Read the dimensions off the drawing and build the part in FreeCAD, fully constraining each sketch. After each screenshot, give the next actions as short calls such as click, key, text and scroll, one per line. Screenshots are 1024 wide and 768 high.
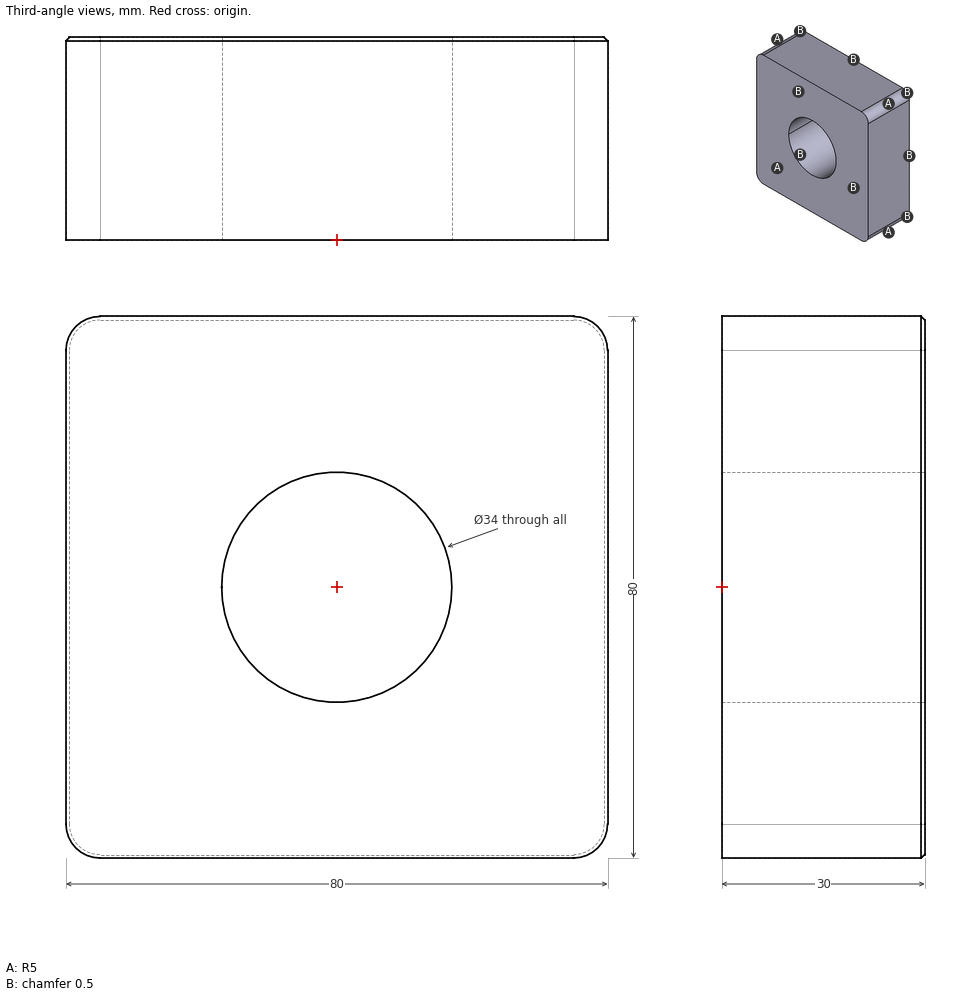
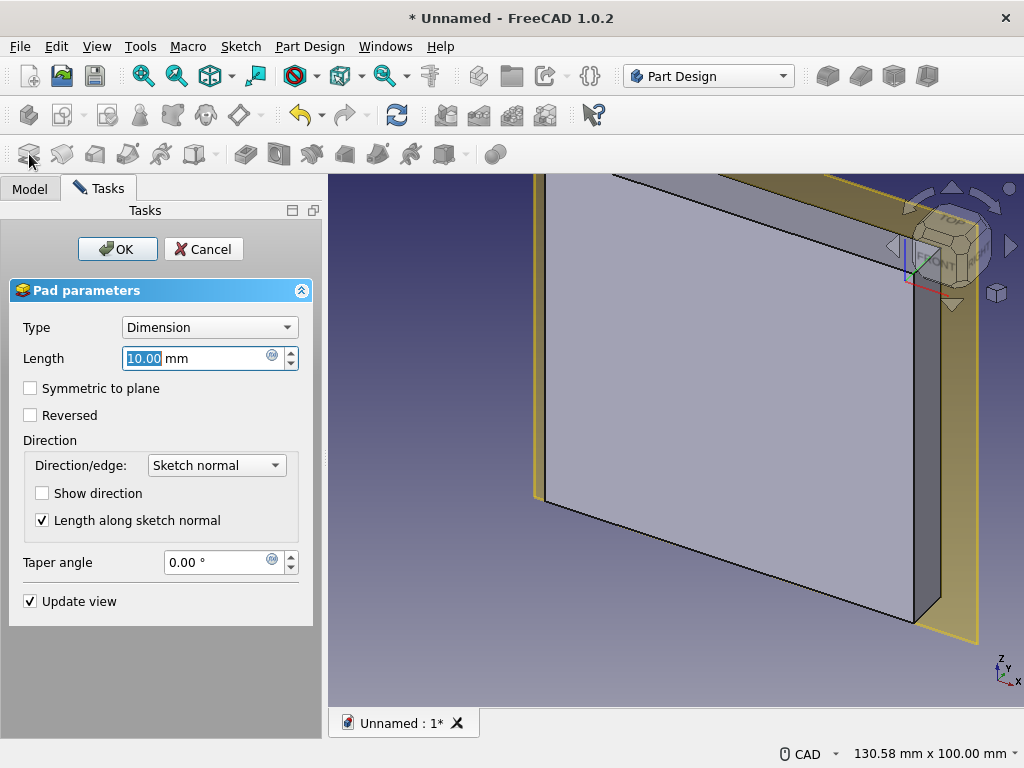
text(30)
key(Tab)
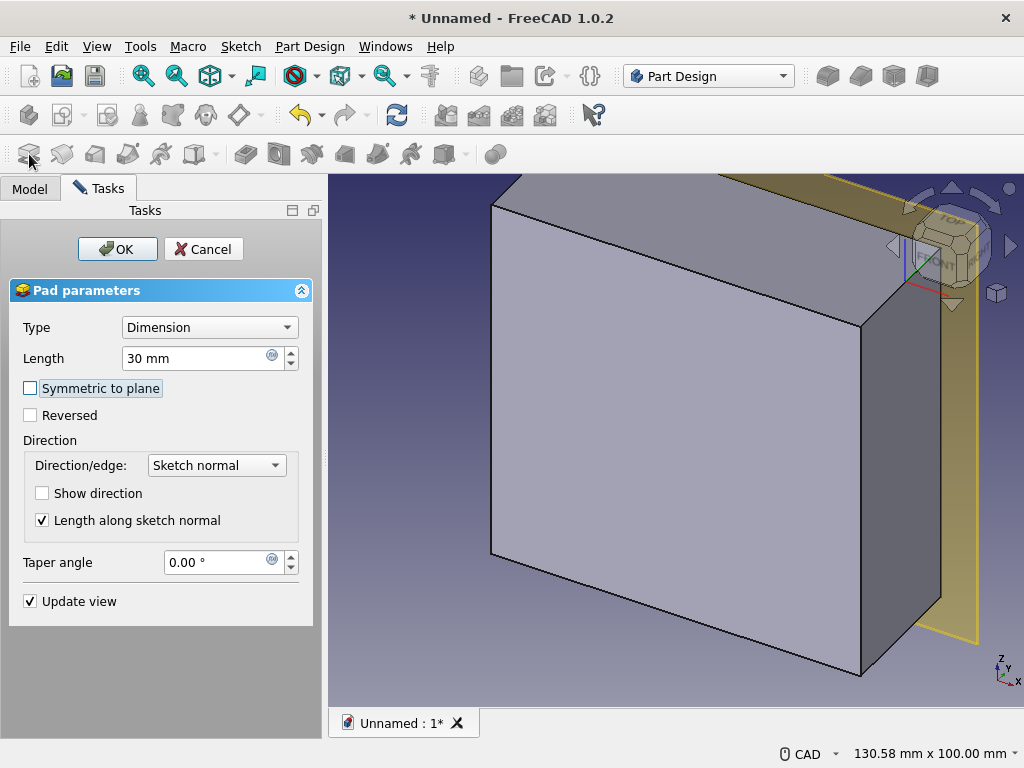
click(118, 249)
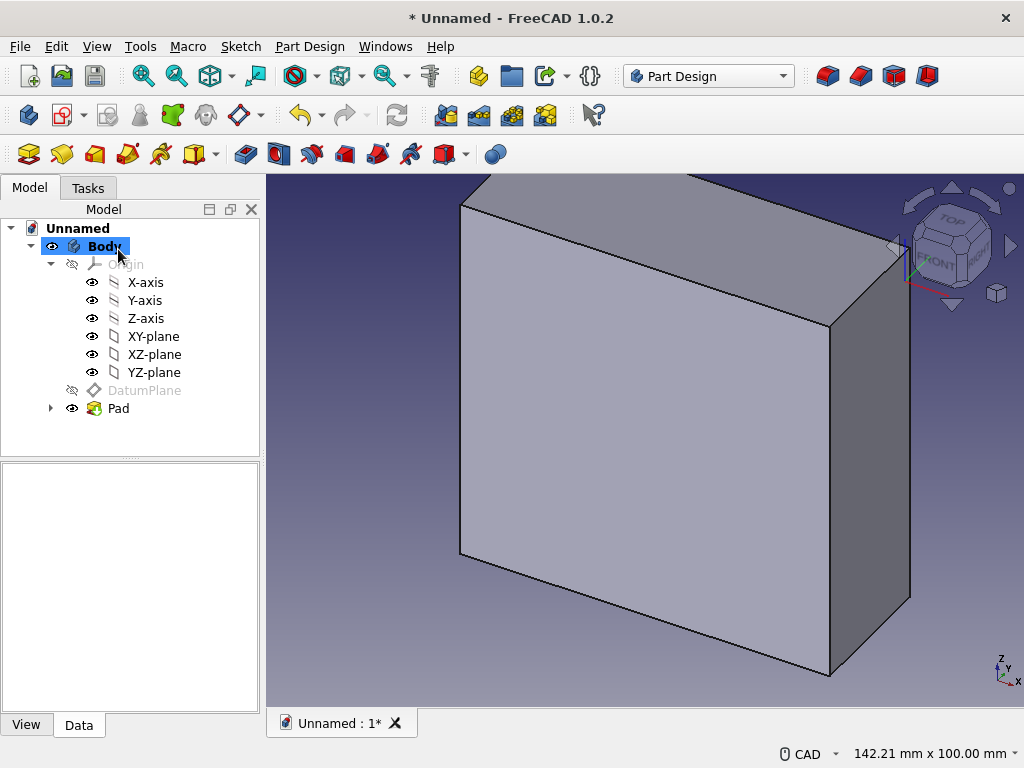
click(144, 76)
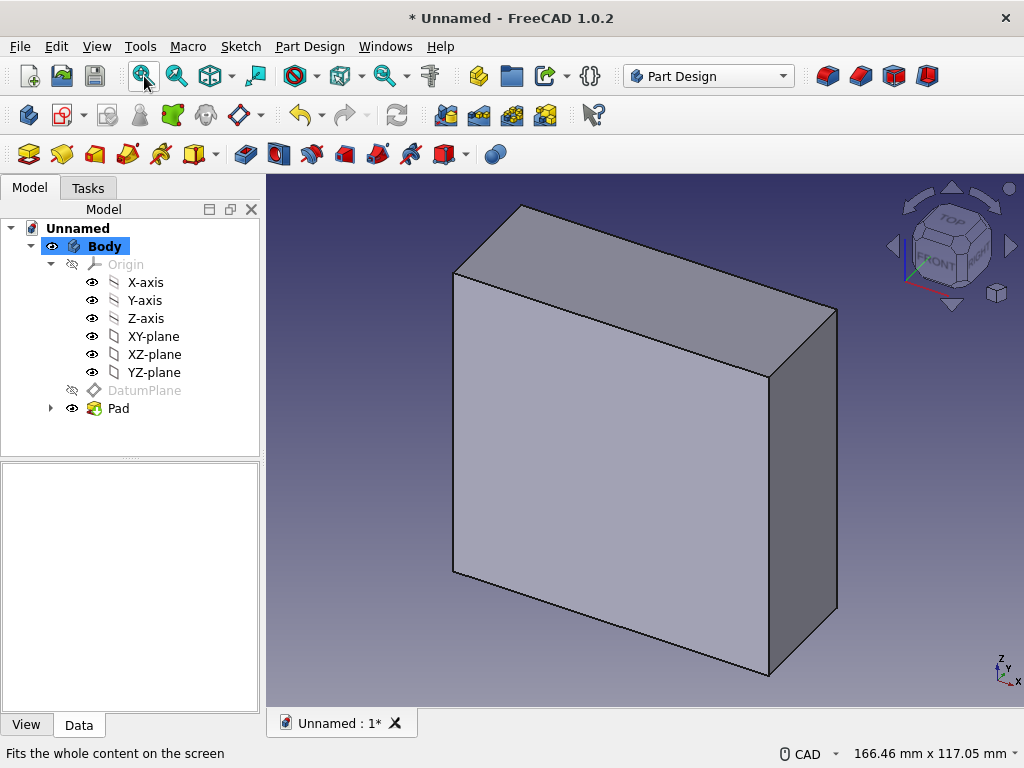
key(4)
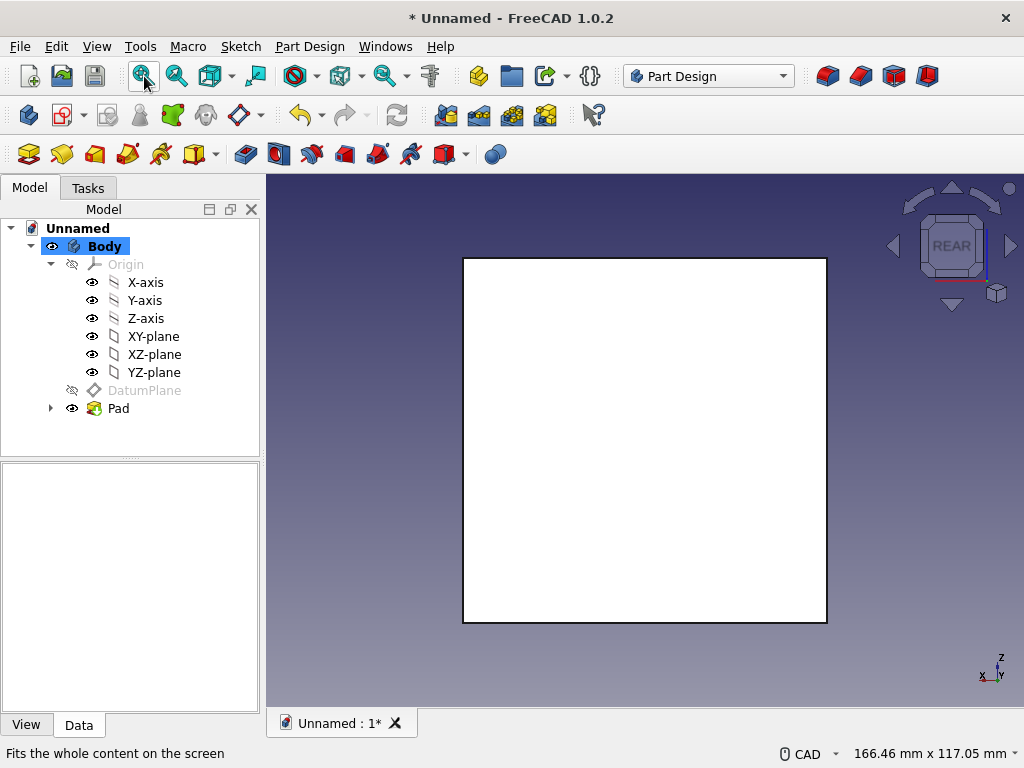
click(645, 440)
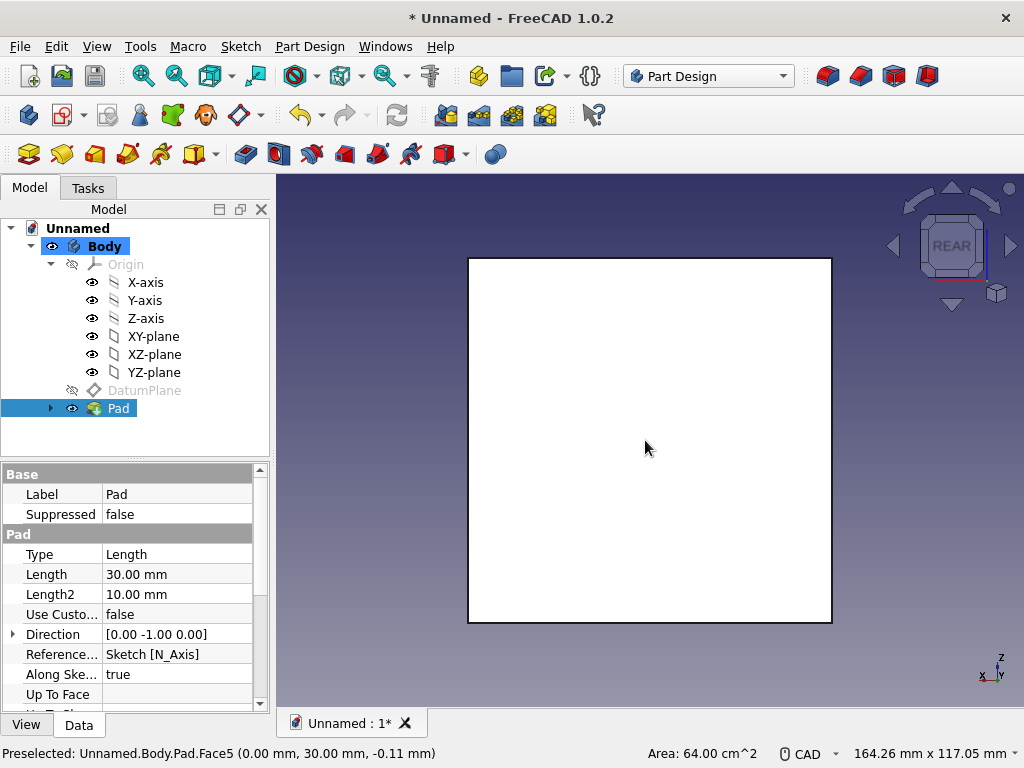
click(62, 116)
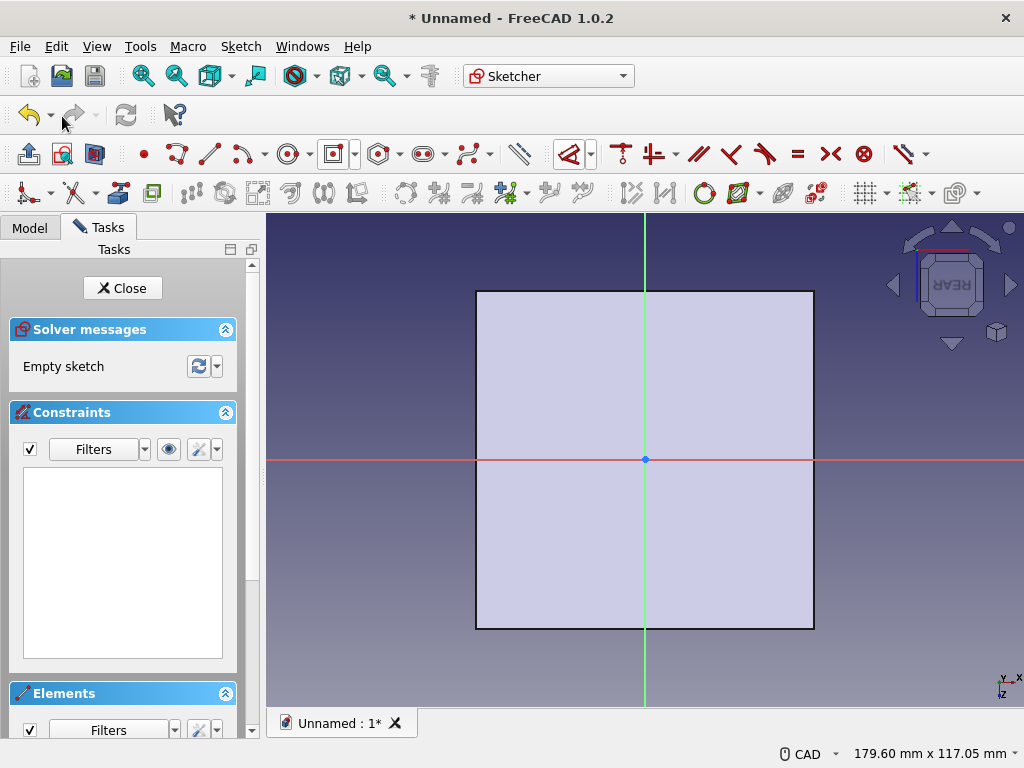
scroll(701, 460, up, 4)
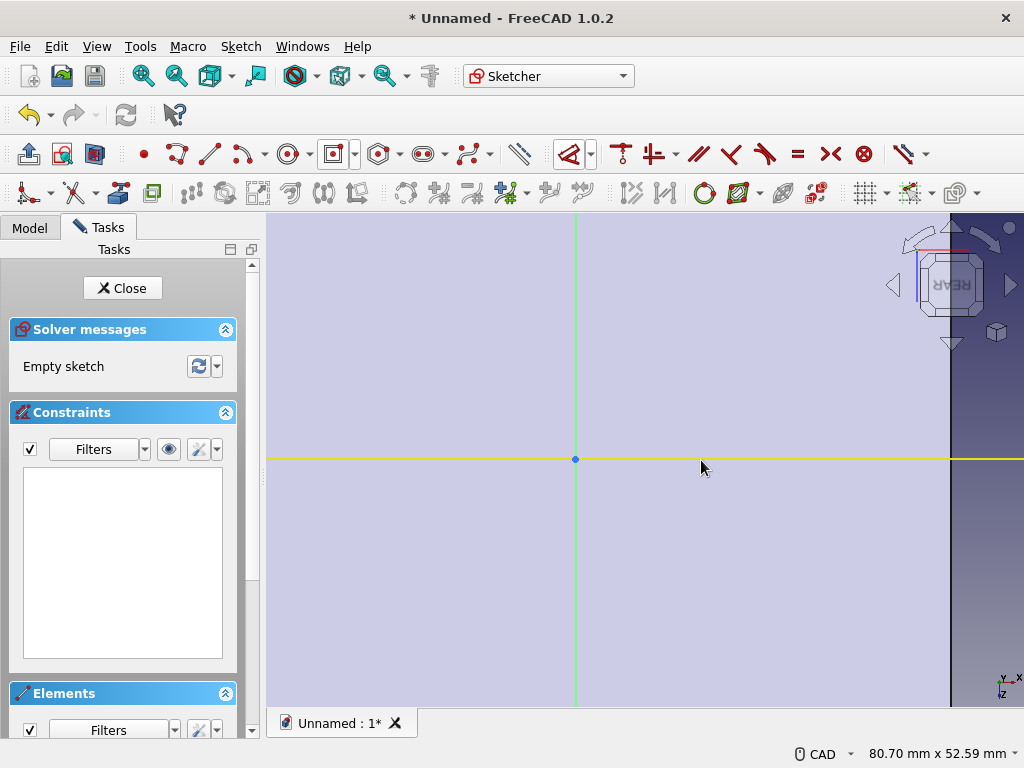
key(g)
key(c)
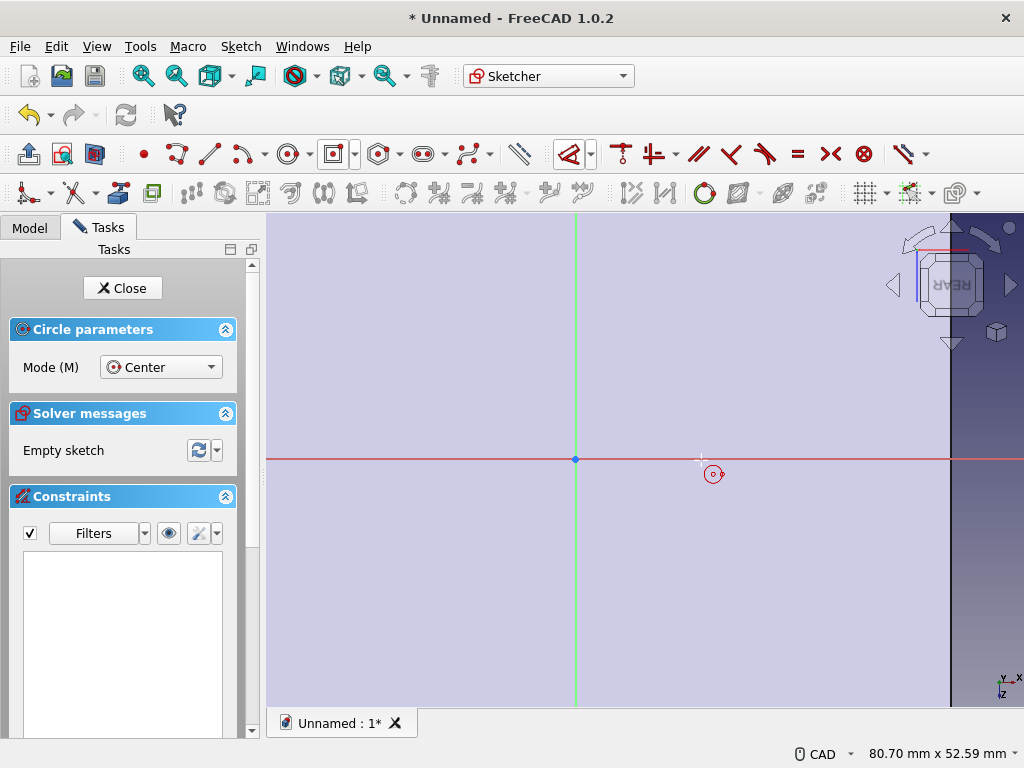
click(576, 459)
click(689, 346)
key(Escape)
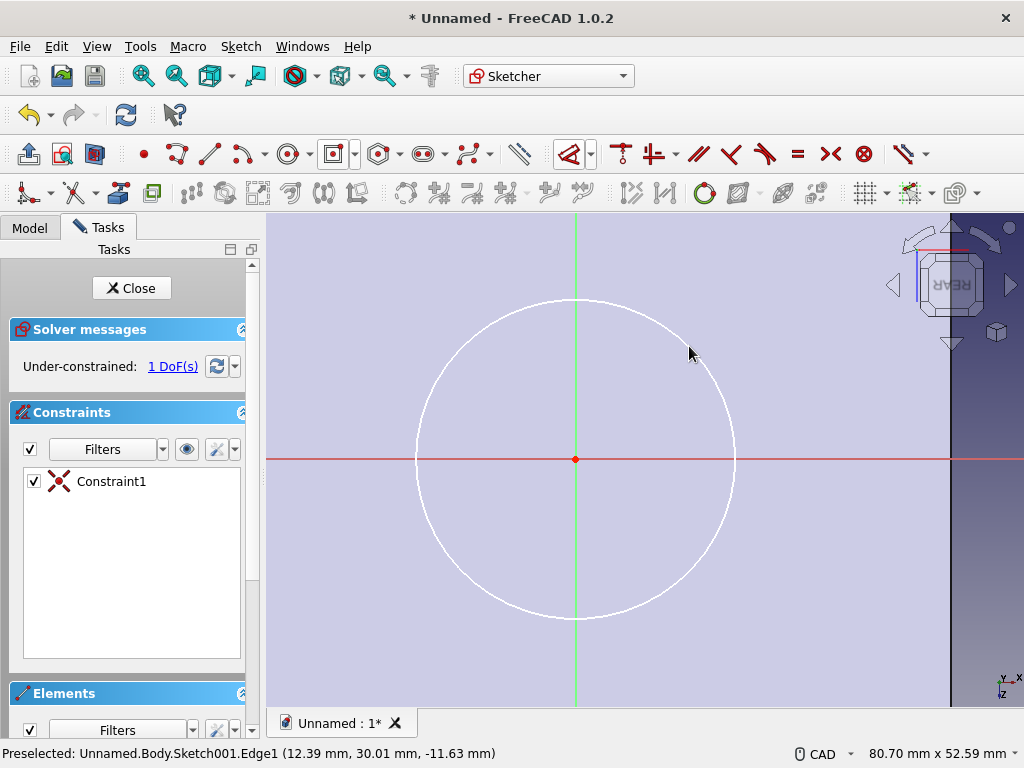
click(688, 346)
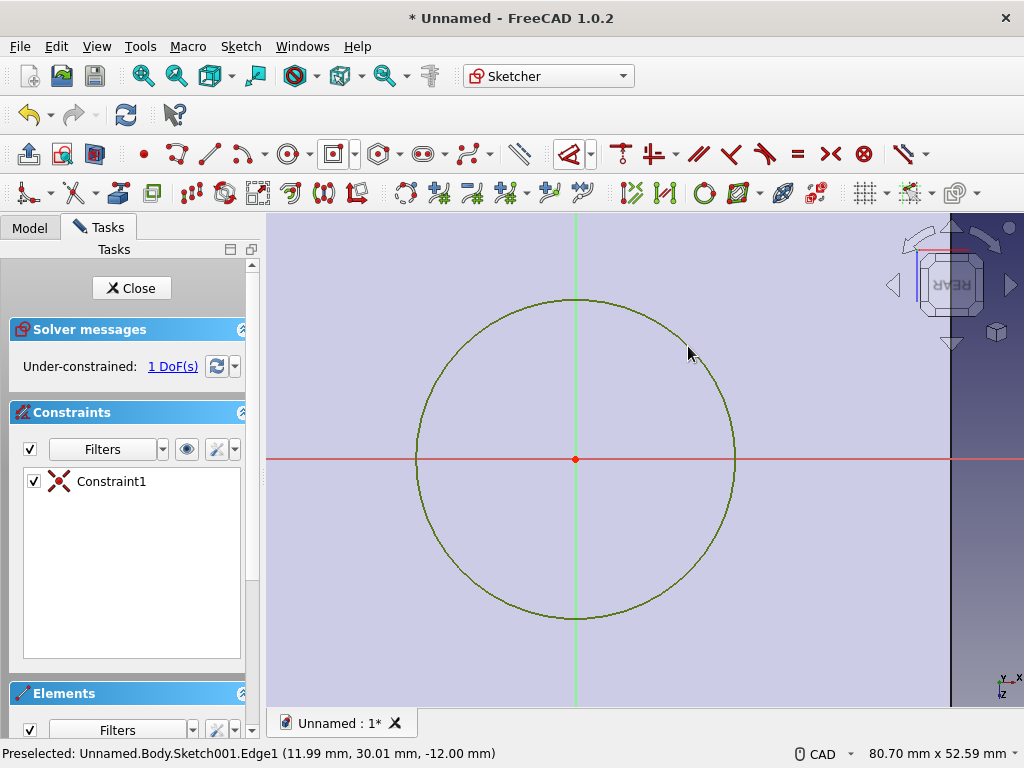
key(k)
key(o)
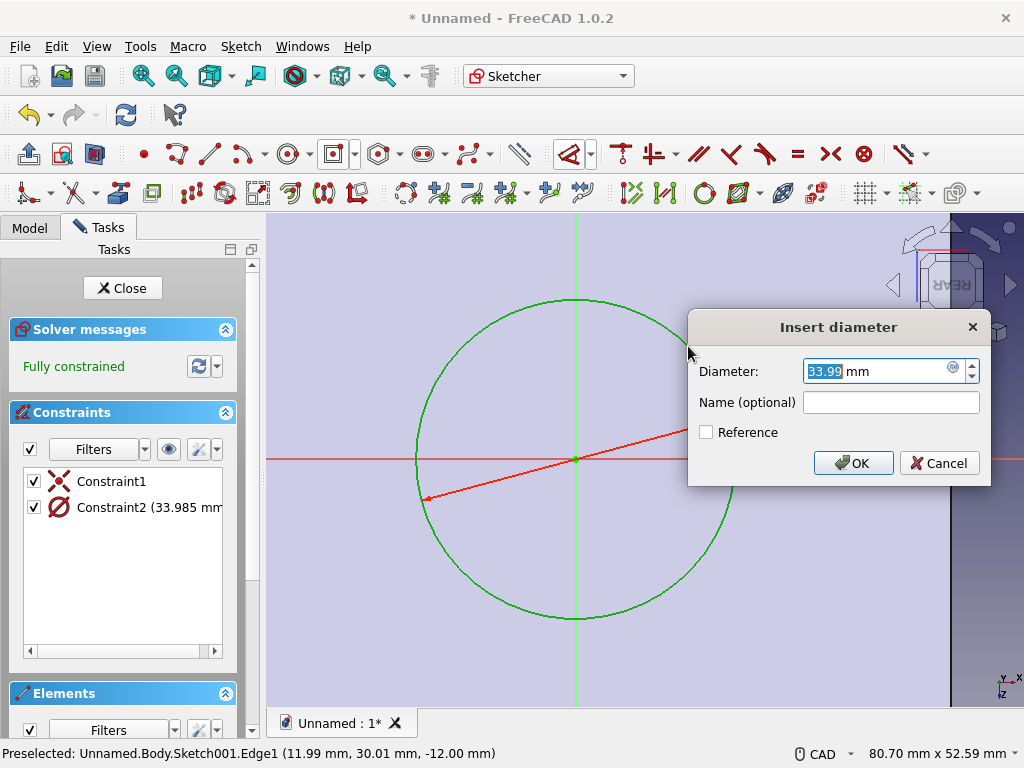
text(34)
key(Return)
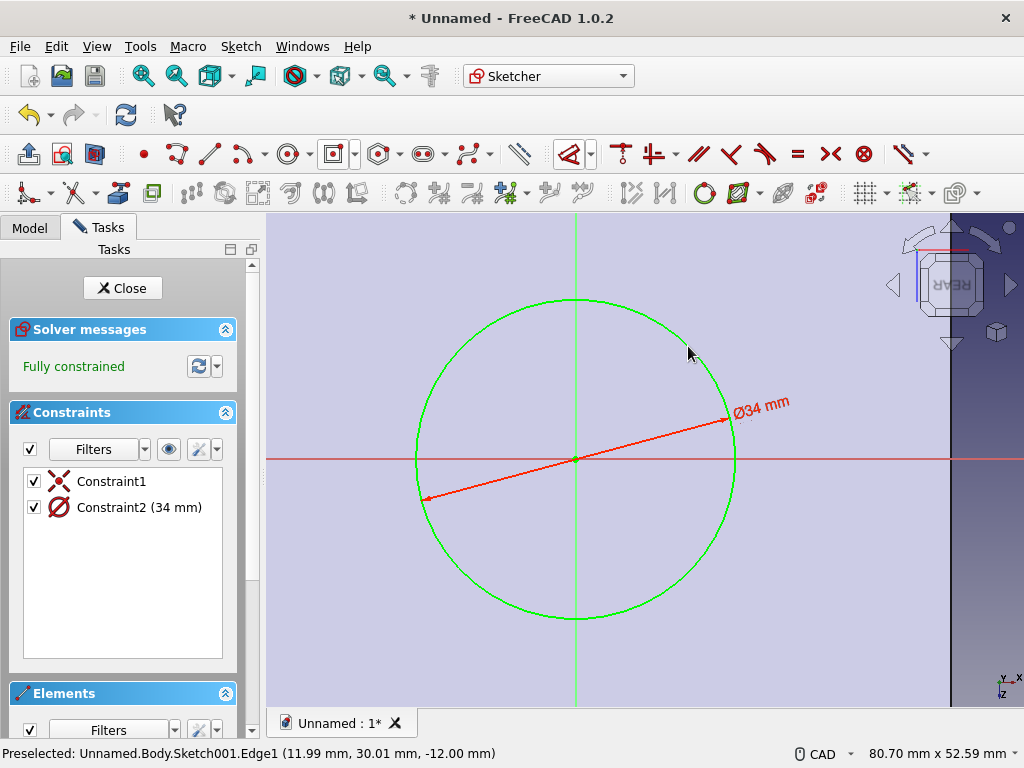
click(123, 288)